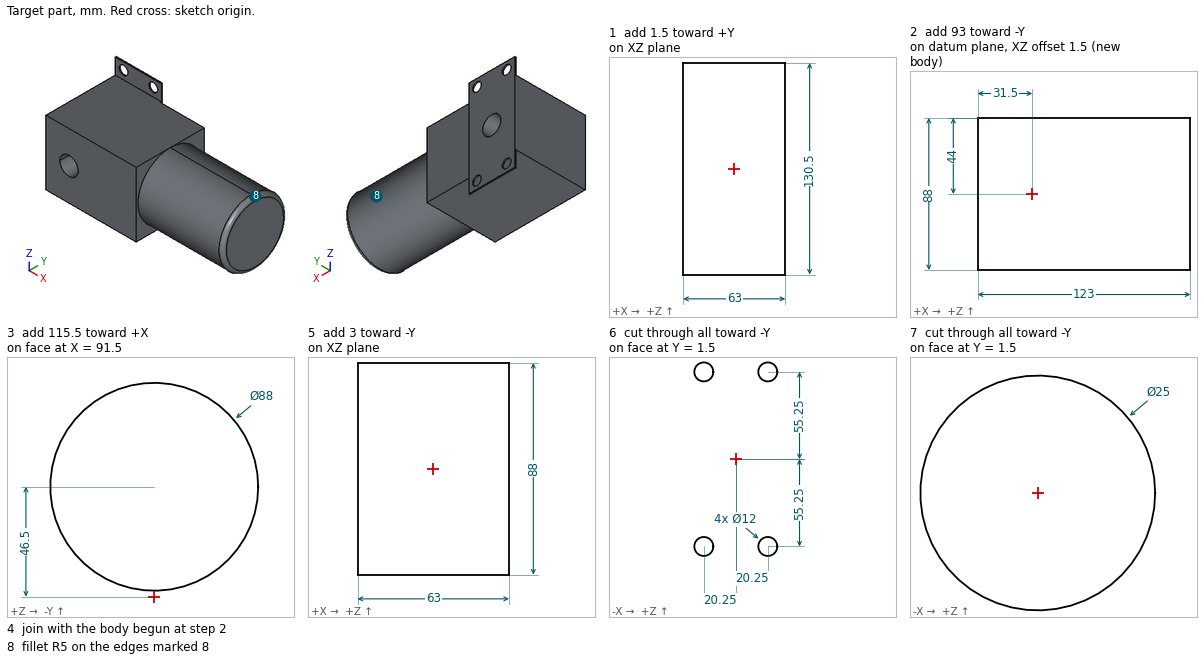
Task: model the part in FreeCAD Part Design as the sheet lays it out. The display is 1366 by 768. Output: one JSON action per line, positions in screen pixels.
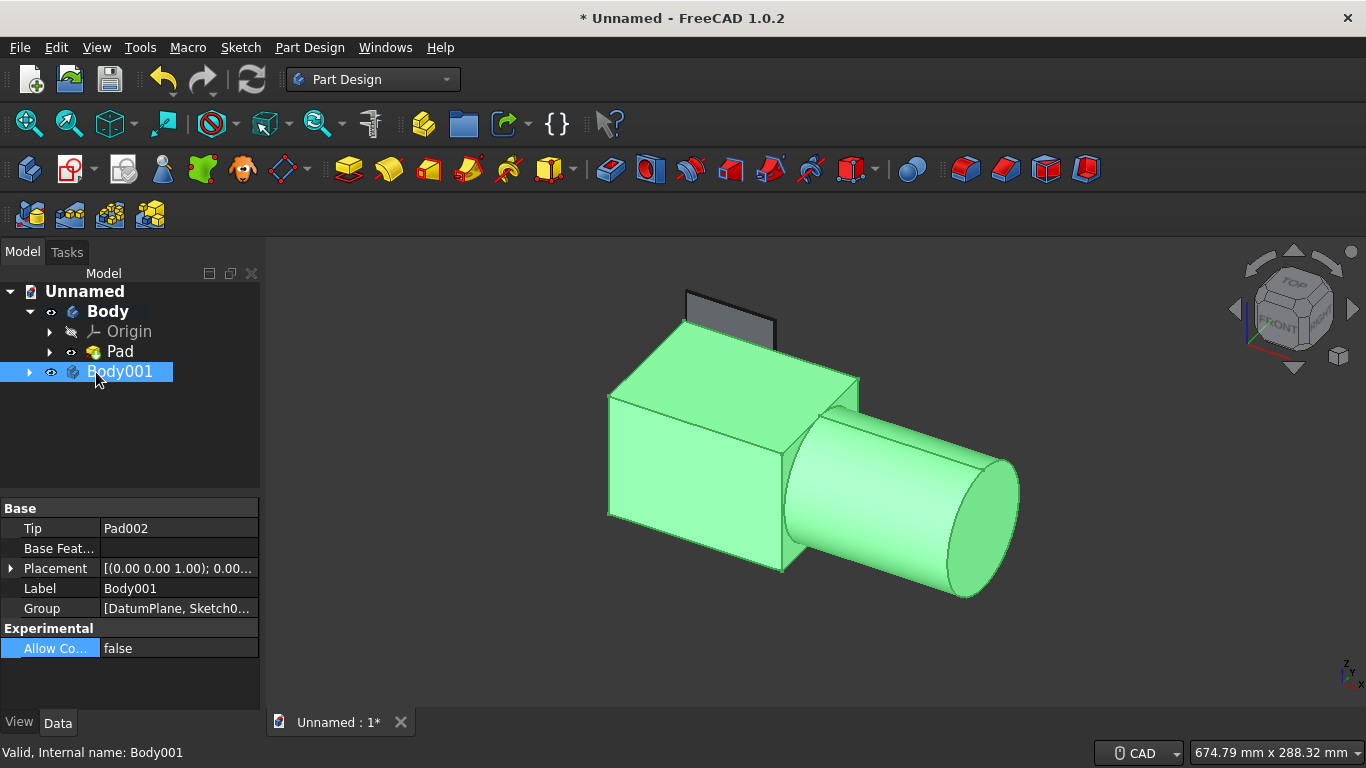
{"action": "left_click", "coordinate": [914, 170]}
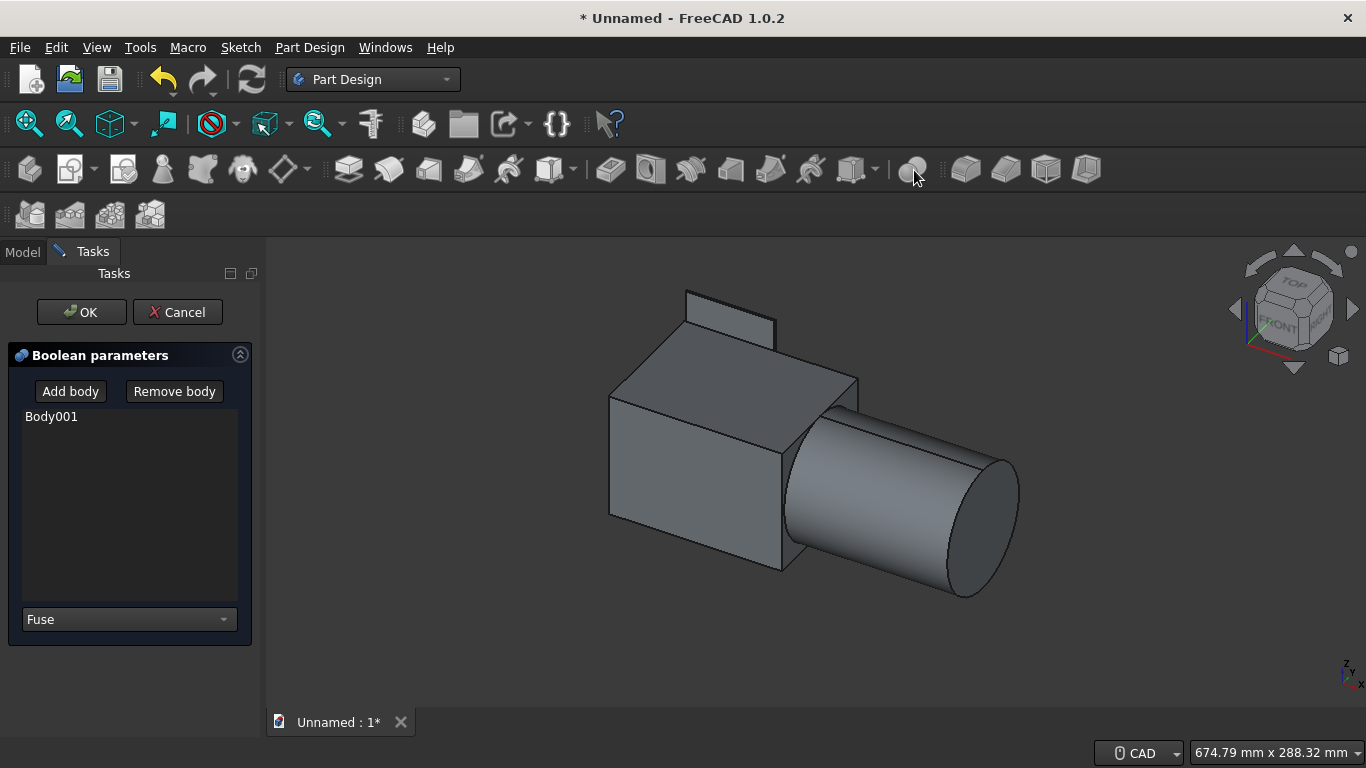
{"action": "left_click", "coordinate": [82, 312]}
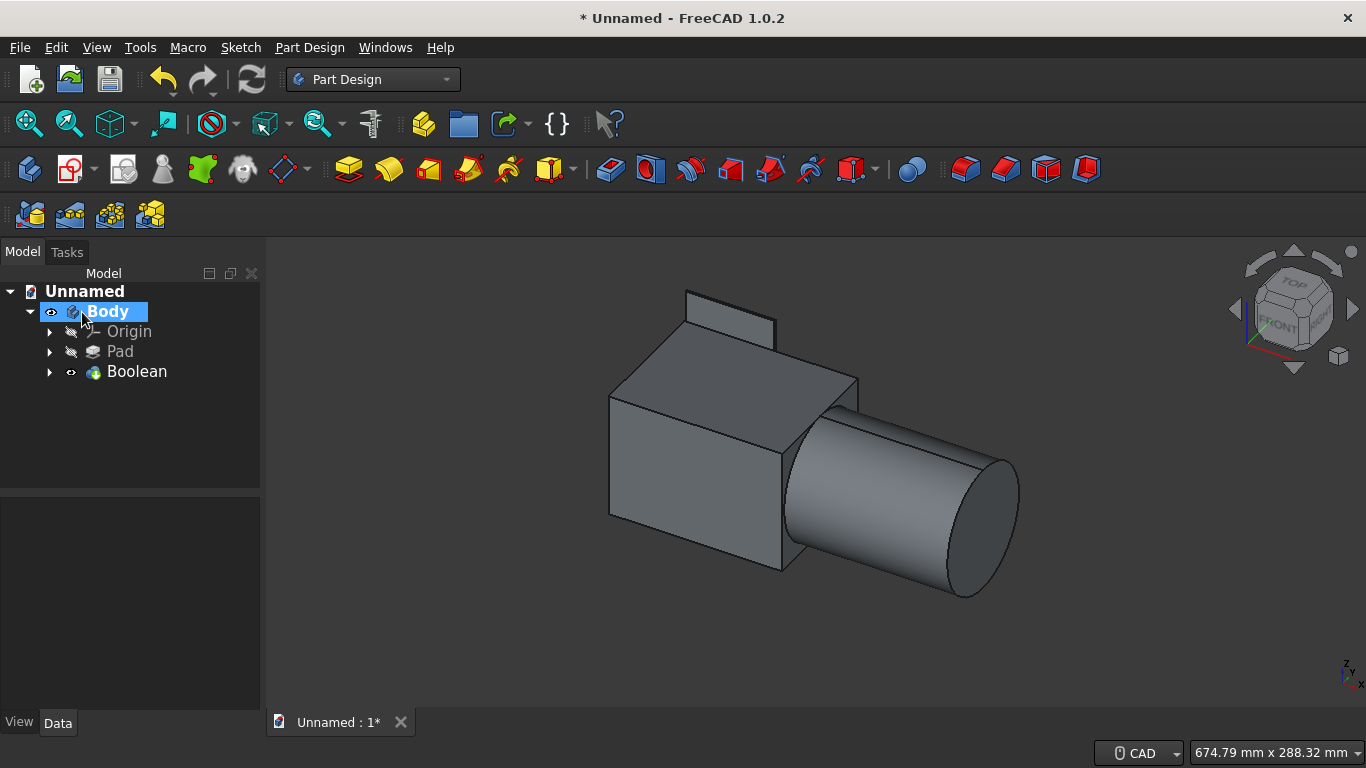
{"action": "left_click", "coordinate": [70, 170]}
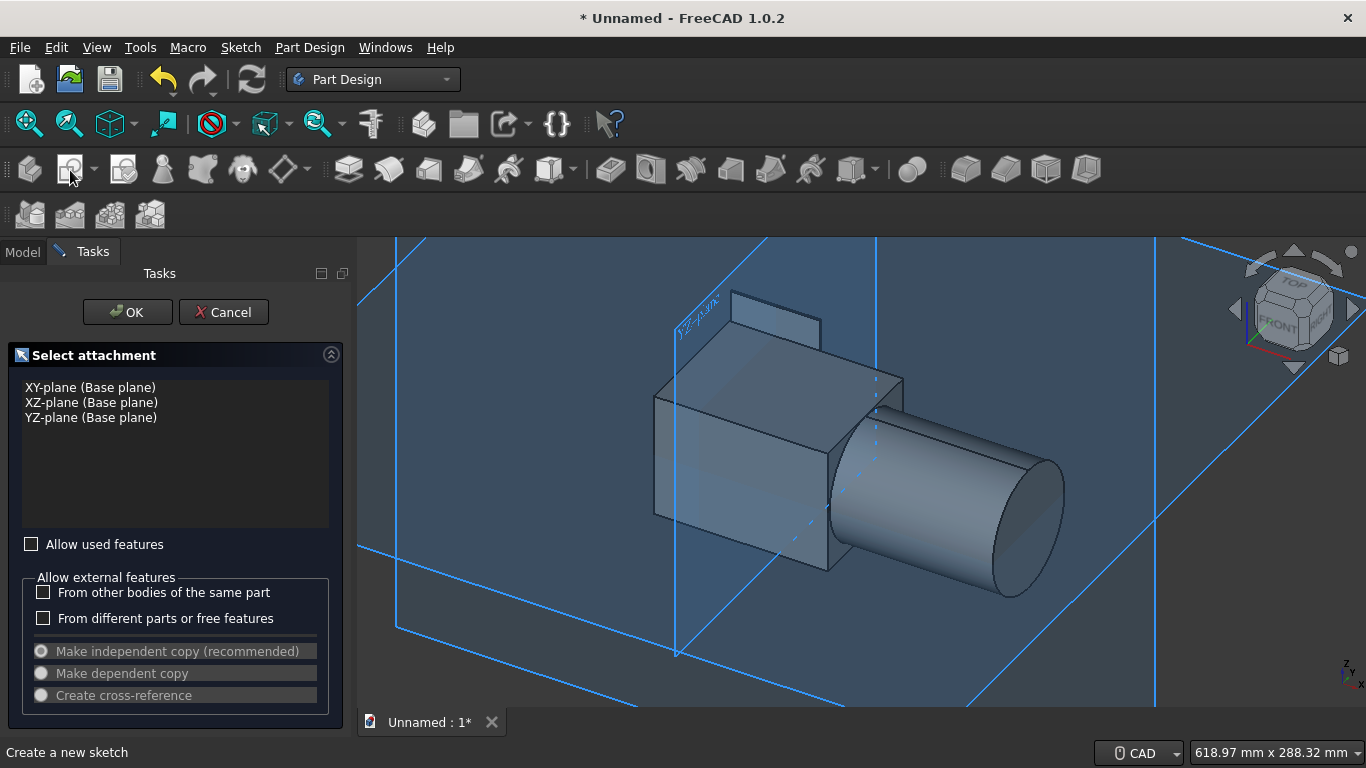
{"action": "left_click", "coordinate": [82, 402]}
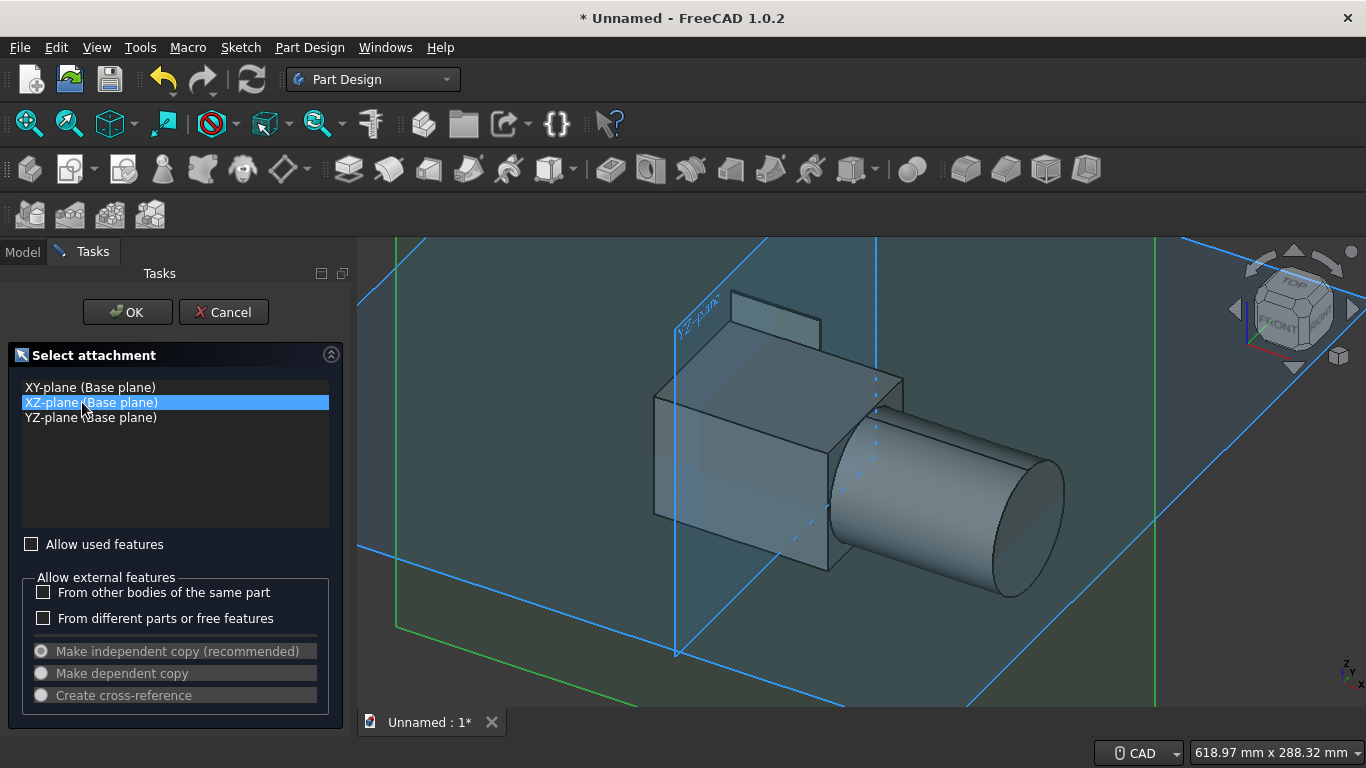
{"action": "left_click", "coordinate": [128, 312]}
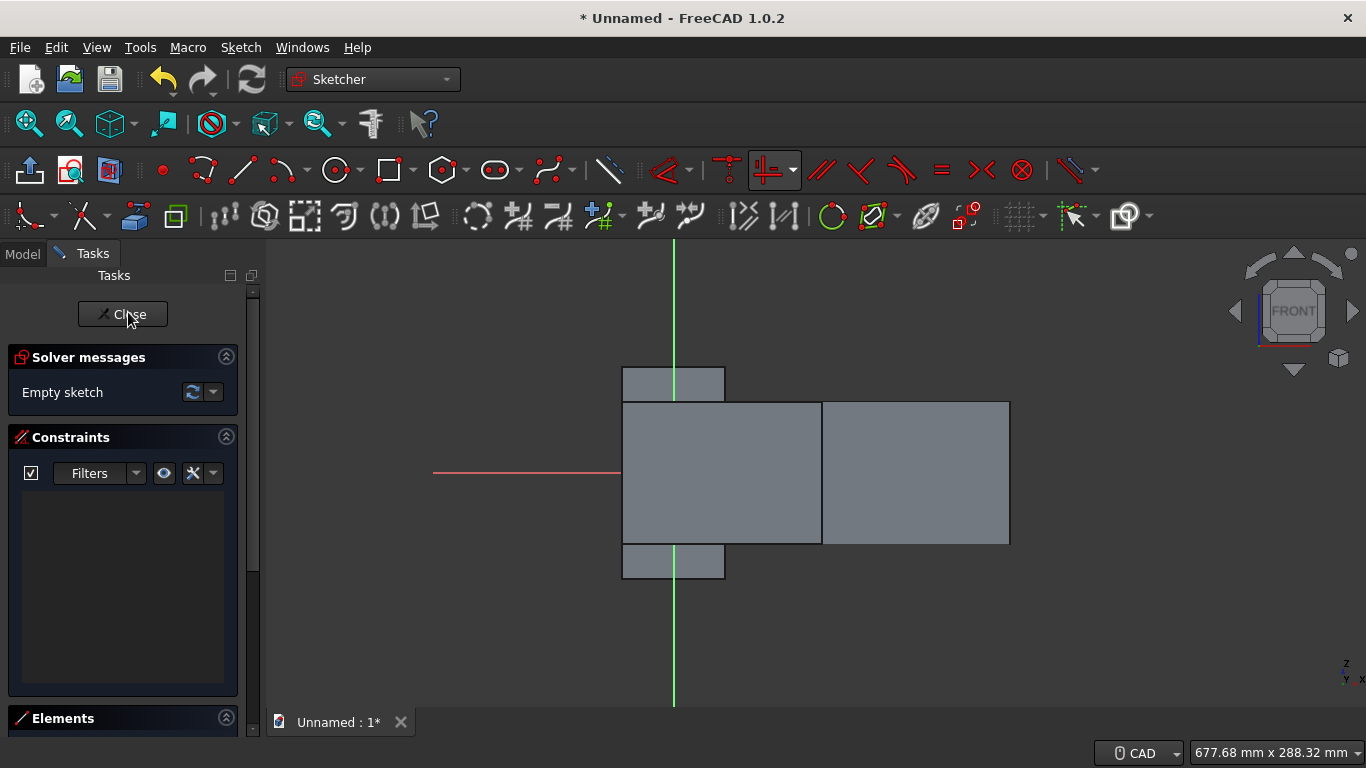
{"action": "left_click", "coordinate": [110, 170]}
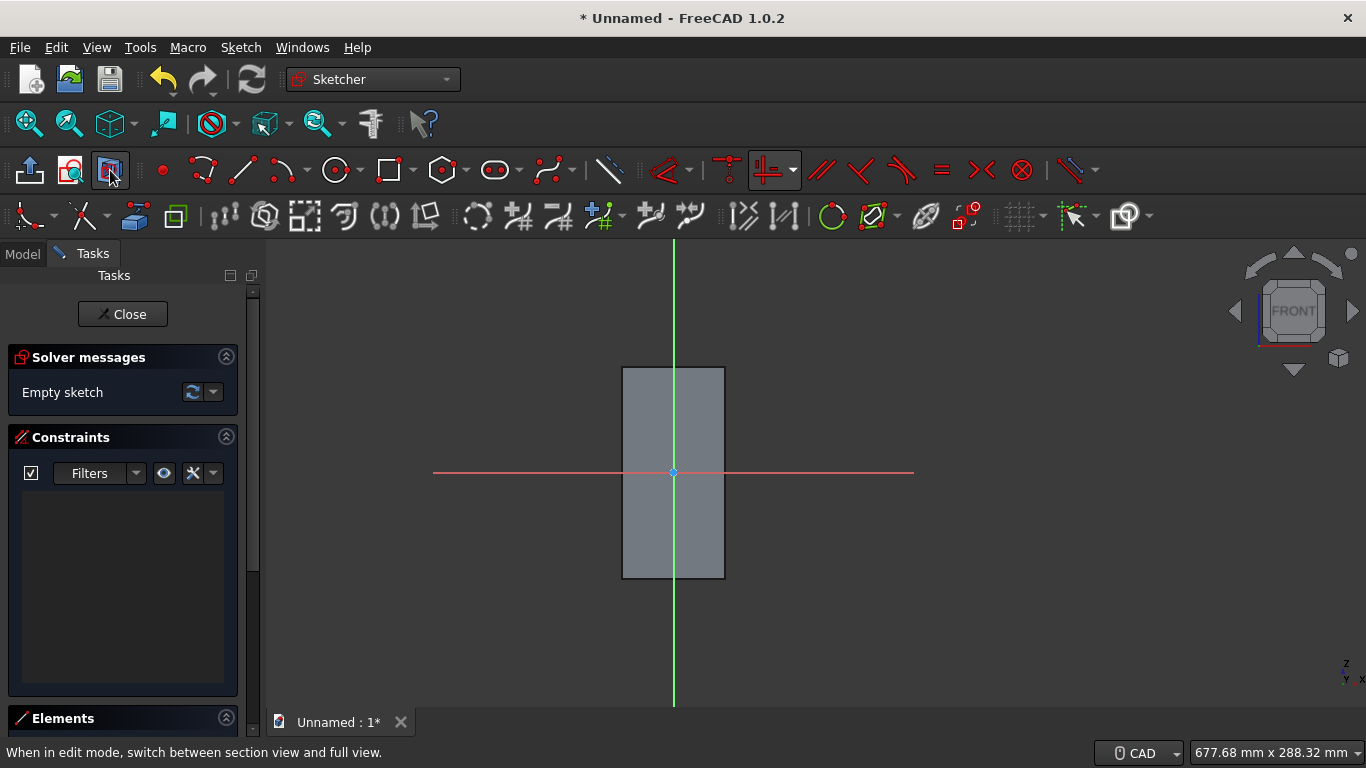
{"action": "scroll", "coordinate": [613, 473], "scroll_direction": "up", "scroll_amount": 4}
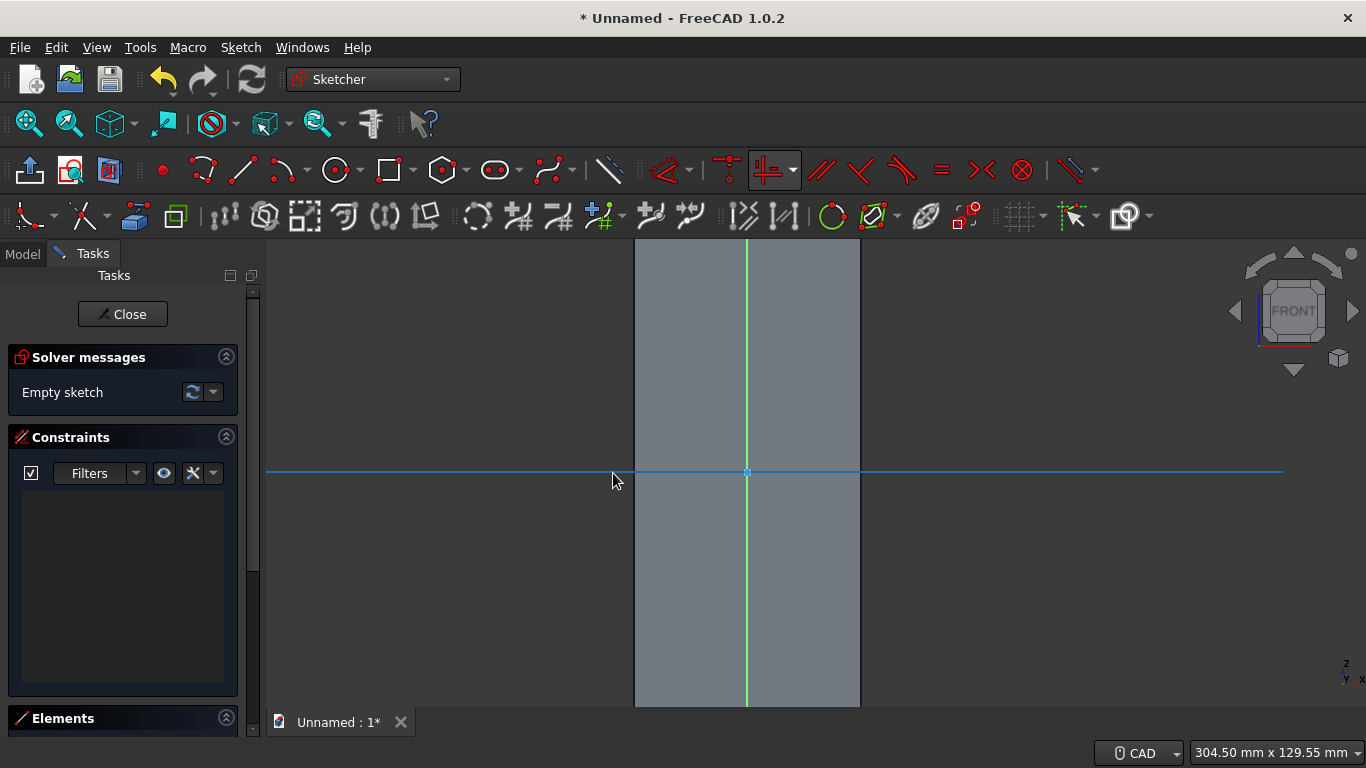
{"action": "left_click", "coordinate": [416, 170]}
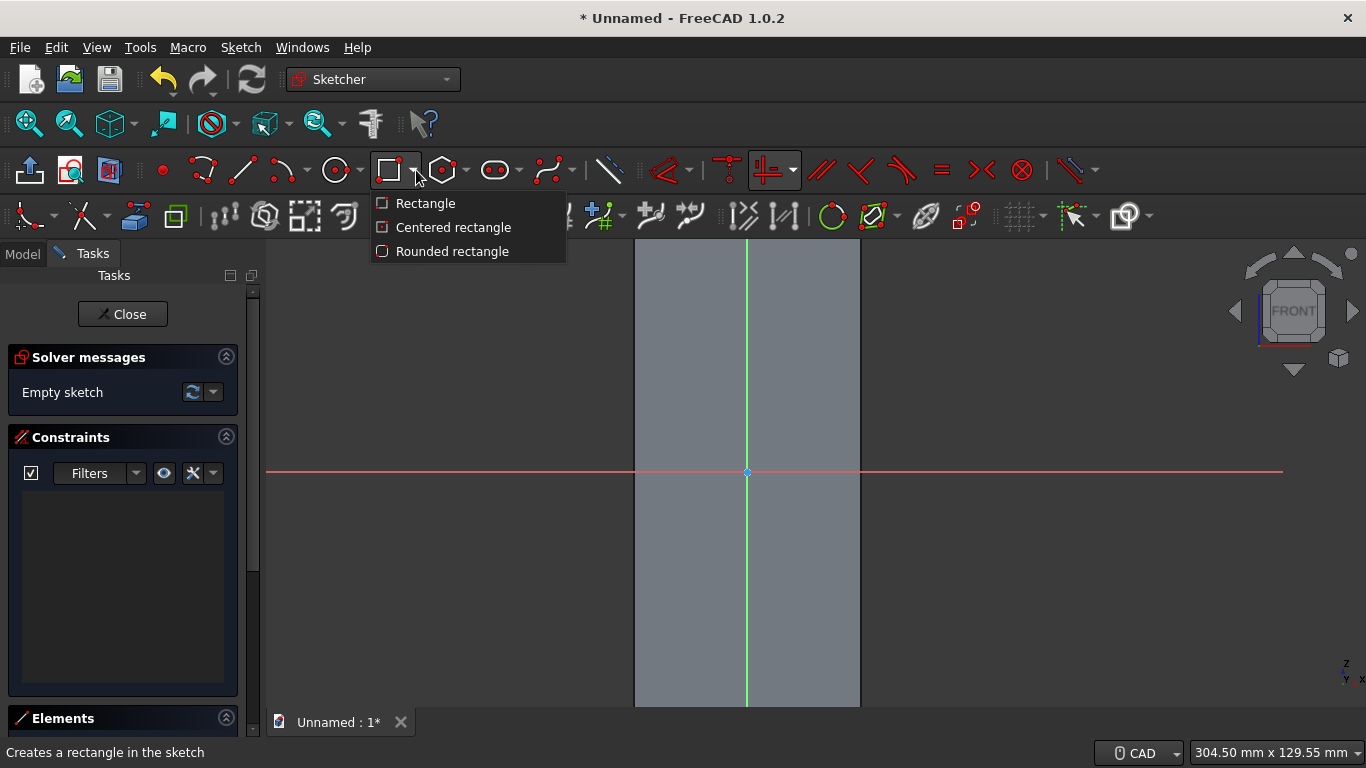
{"action": "left_click", "coordinate": [468, 227]}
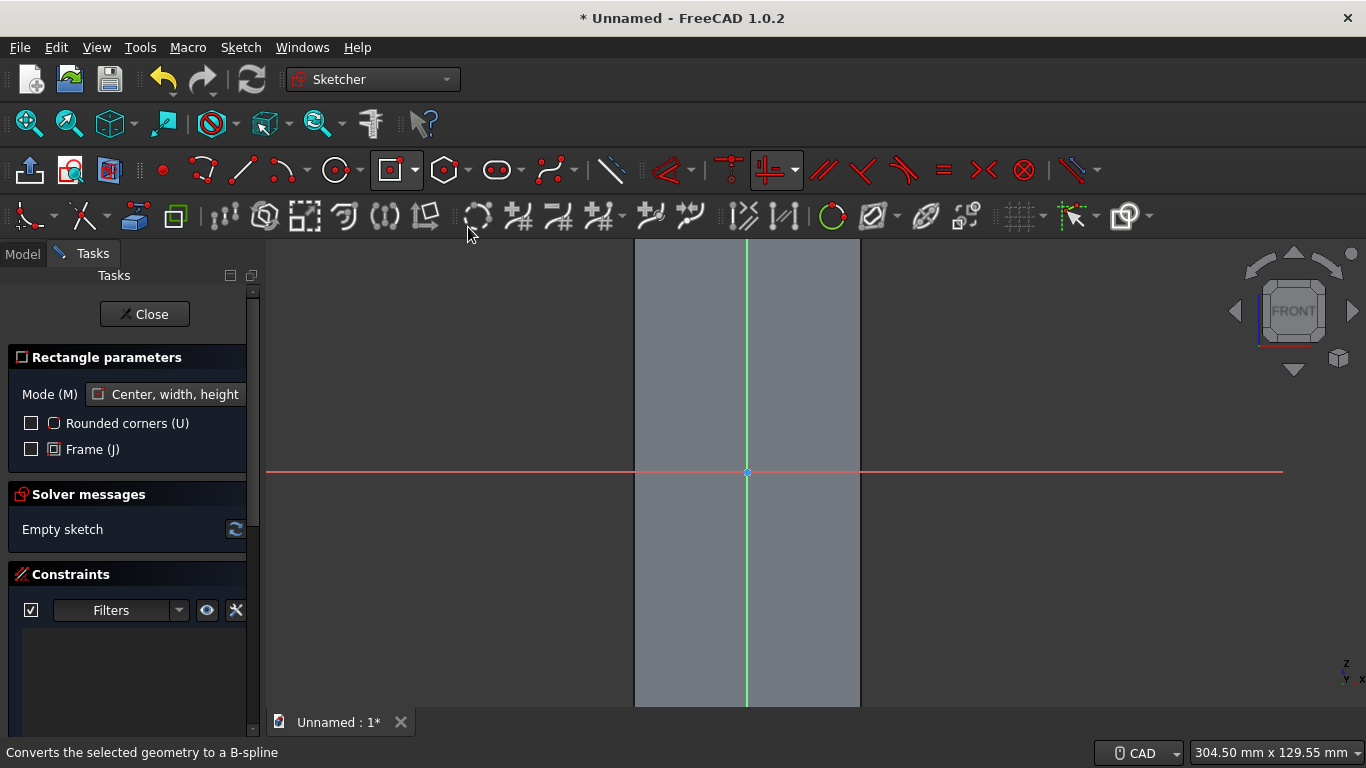
{"action": "left_click", "coordinate": [747, 472]}
{"action": "left_click", "coordinate": [861, 313]}
{"action": "key", "text": "Escape"}